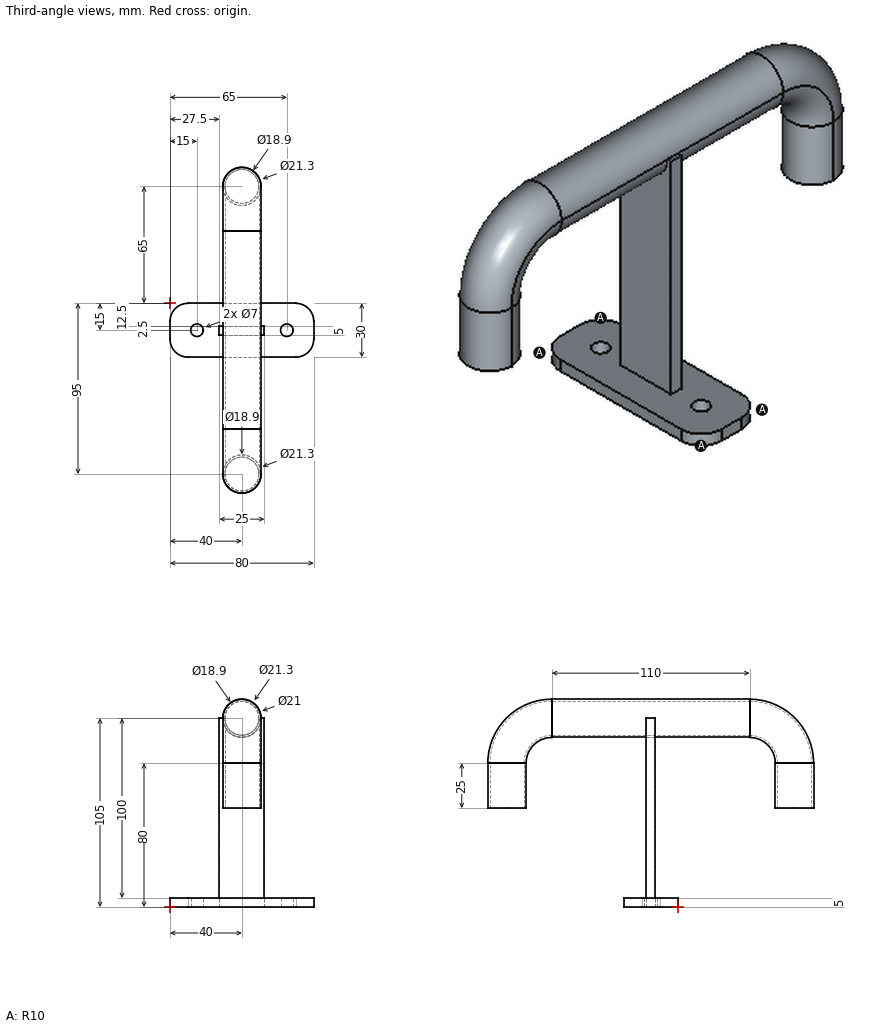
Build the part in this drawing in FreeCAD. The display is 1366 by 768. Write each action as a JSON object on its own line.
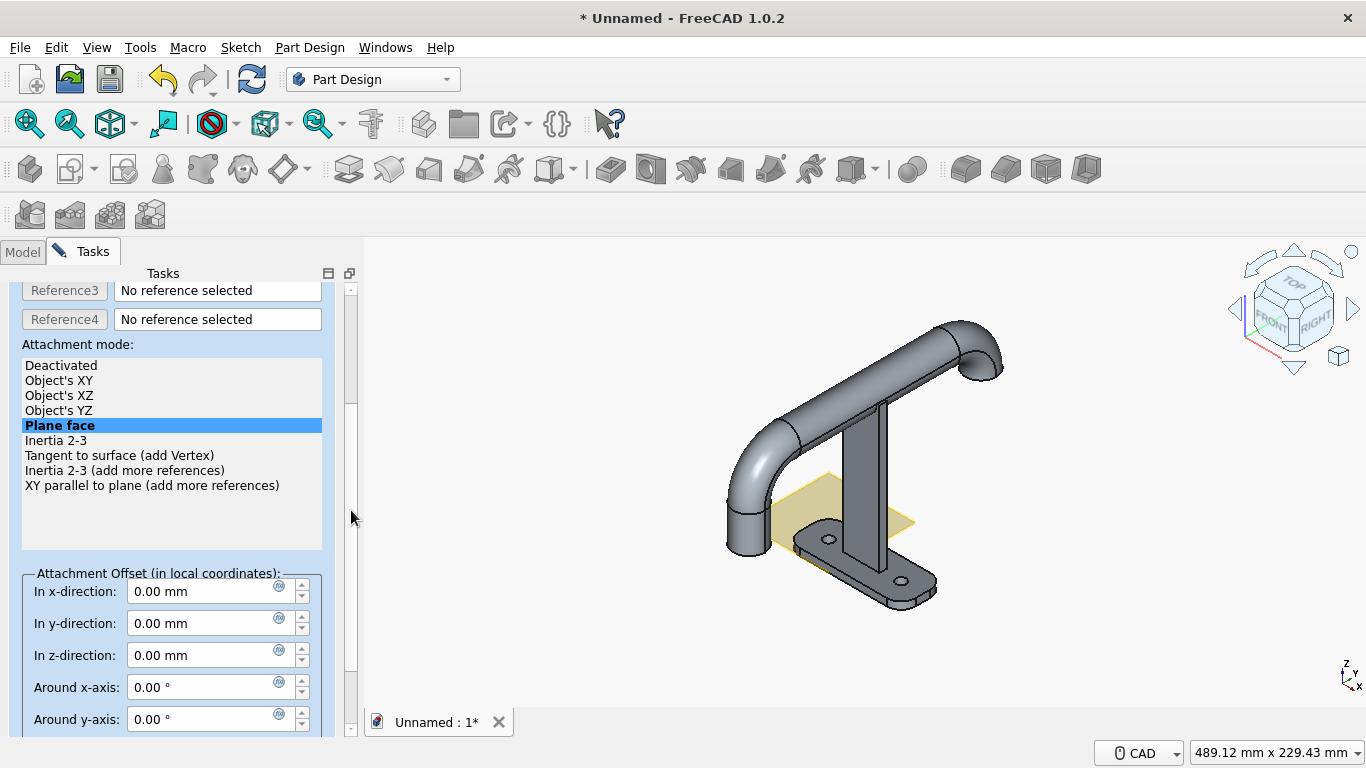
{"action": "triple_click", "coordinate": [210, 655]}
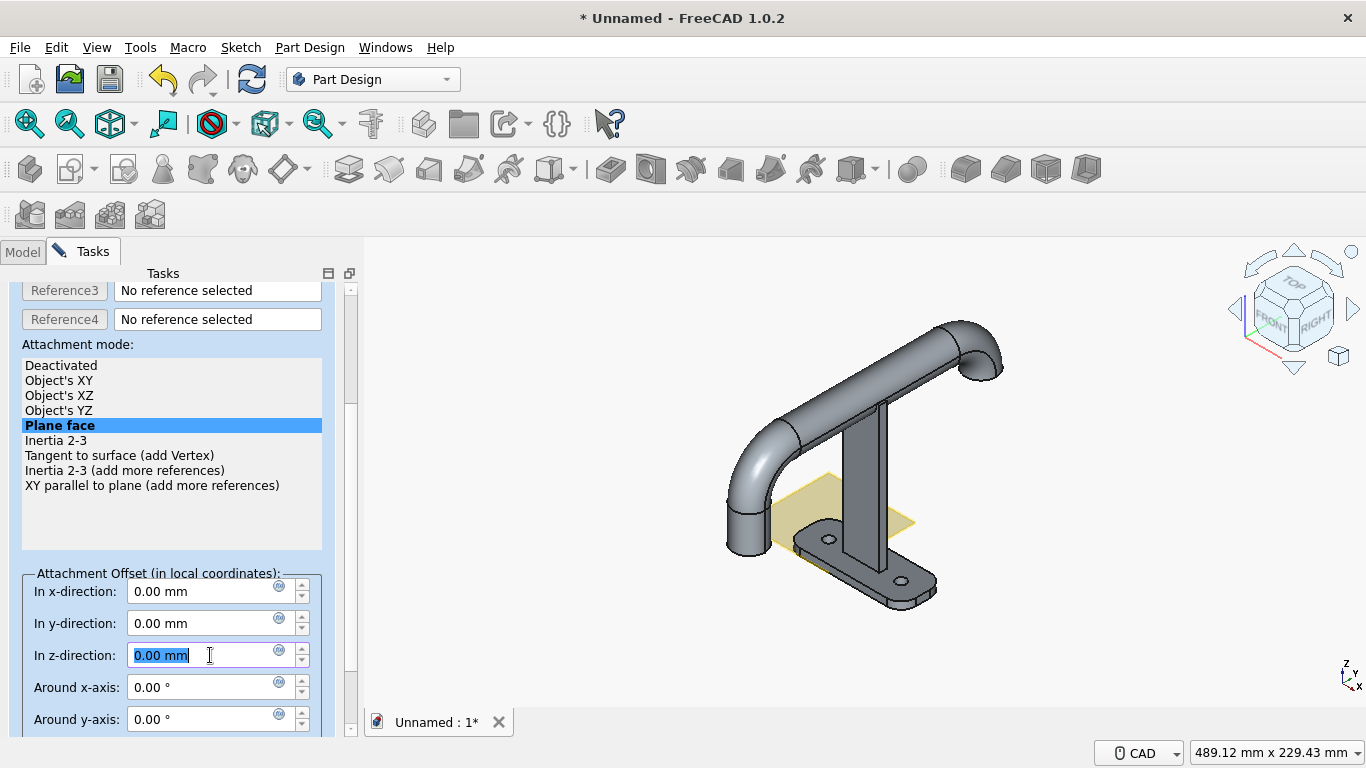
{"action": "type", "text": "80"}
{"action": "key", "text": "Tab"}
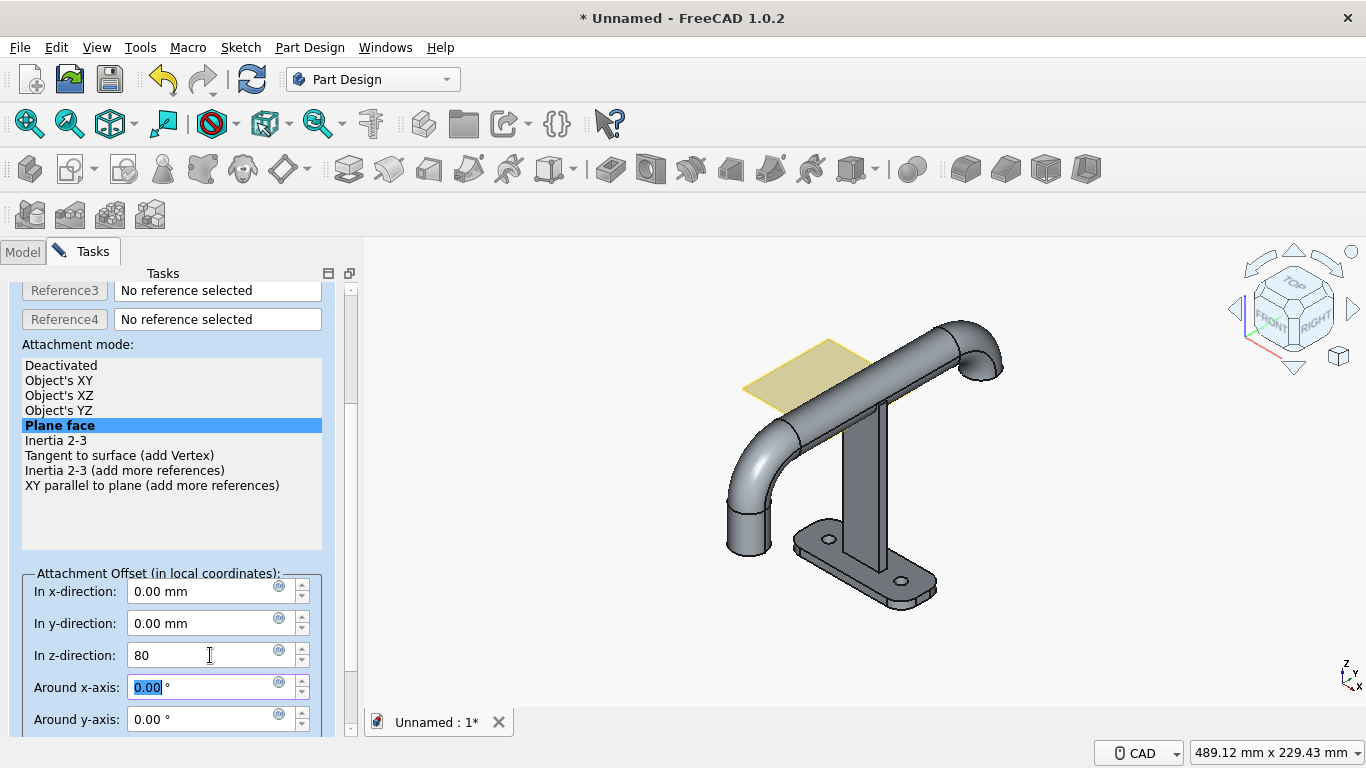
{"action": "scroll", "coordinate": [351, 510], "scroll_direction": "up", "scroll_amount": 4}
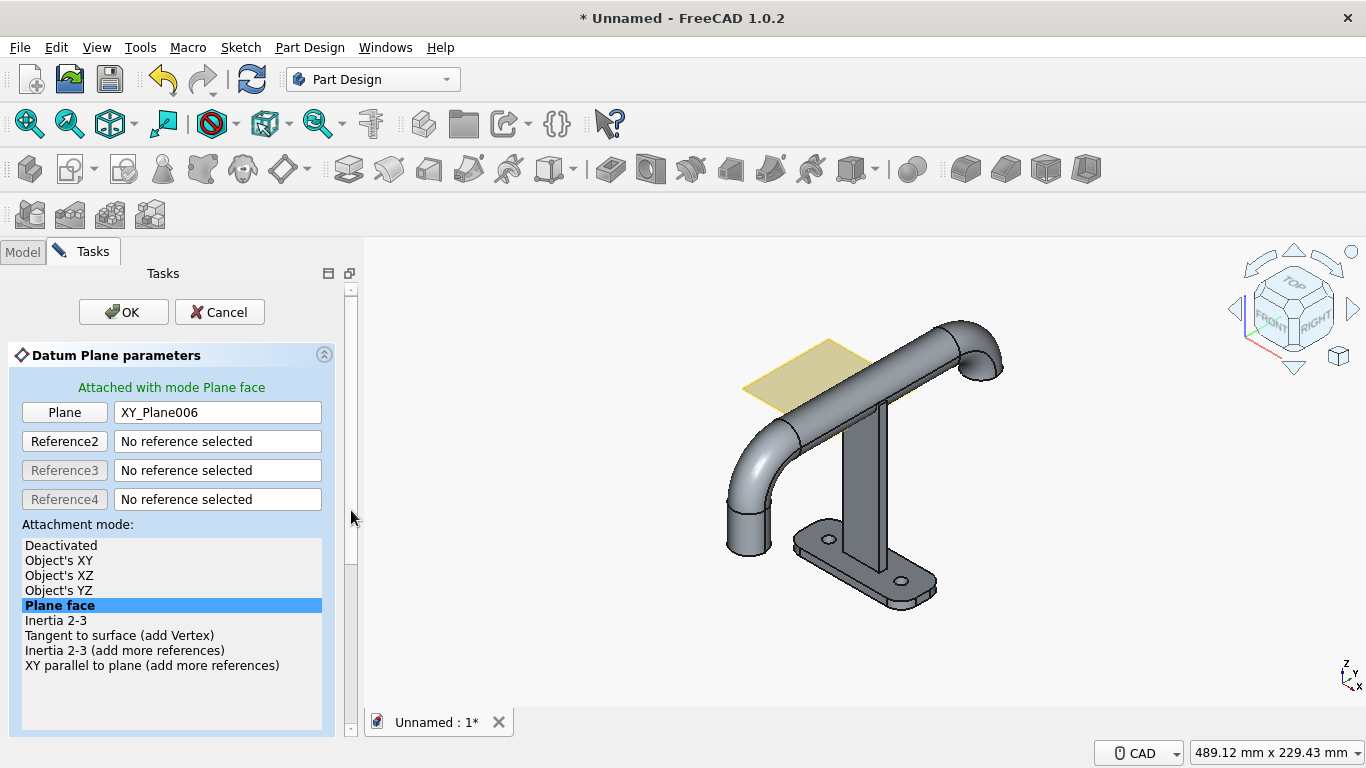
{"action": "left_click", "coordinate": [124, 312]}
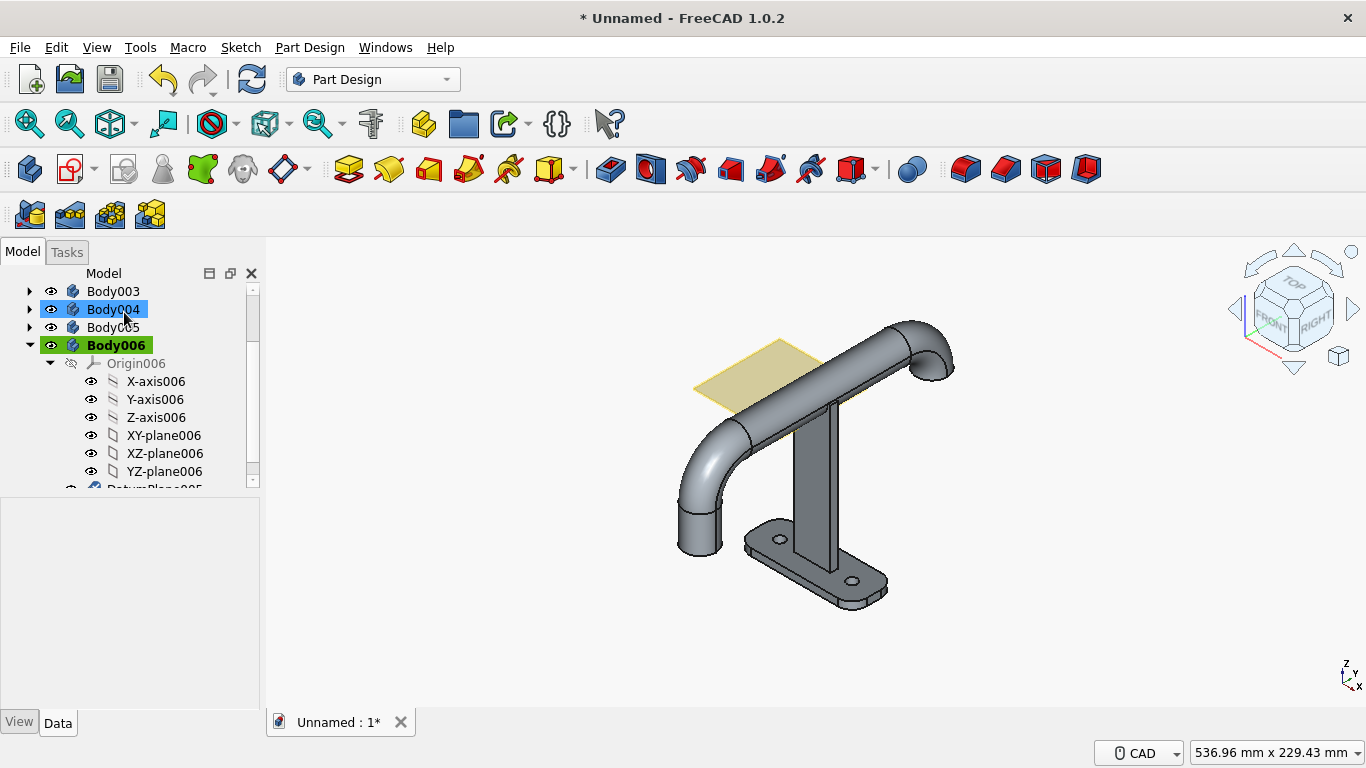
{"action": "scroll", "coordinate": [120, 377], "scroll_direction": "down", "scroll_amount": 3}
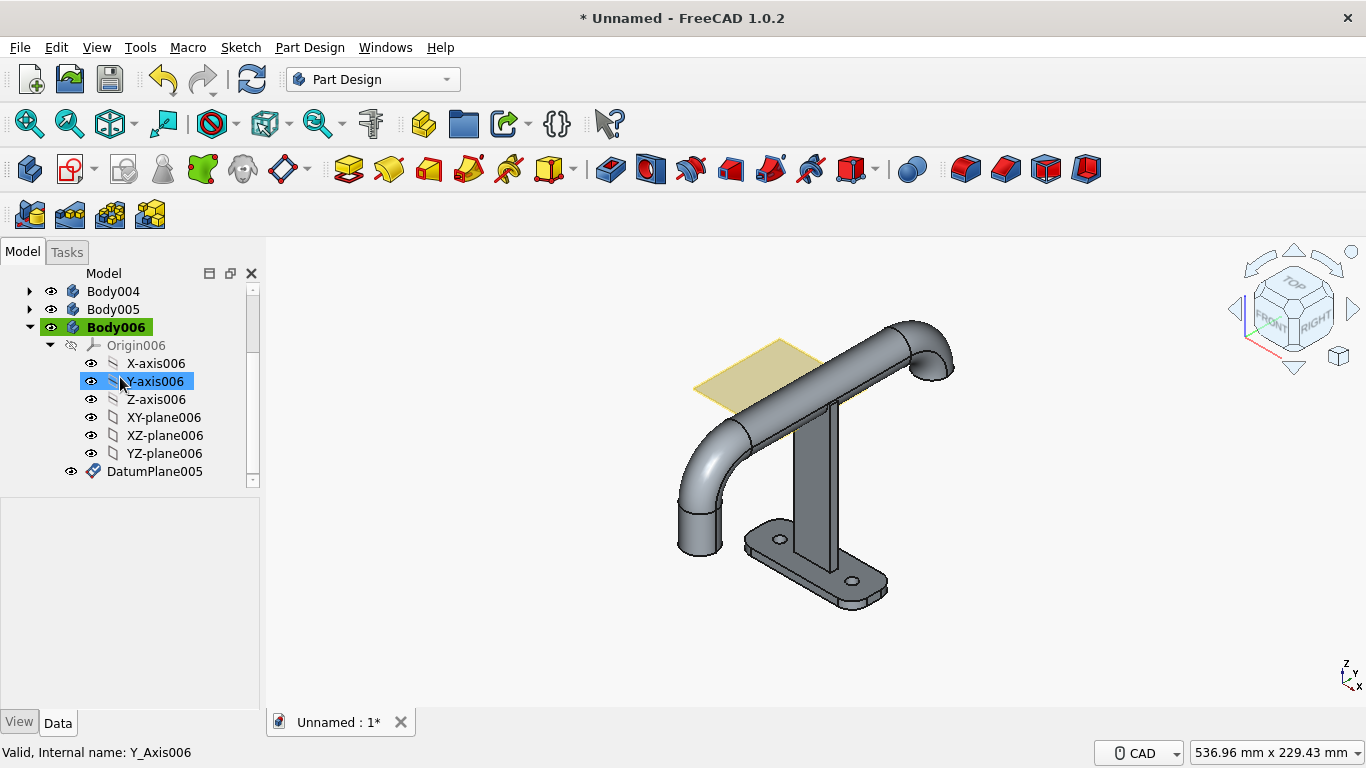
{"action": "left_click", "coordinate": [116, 471]}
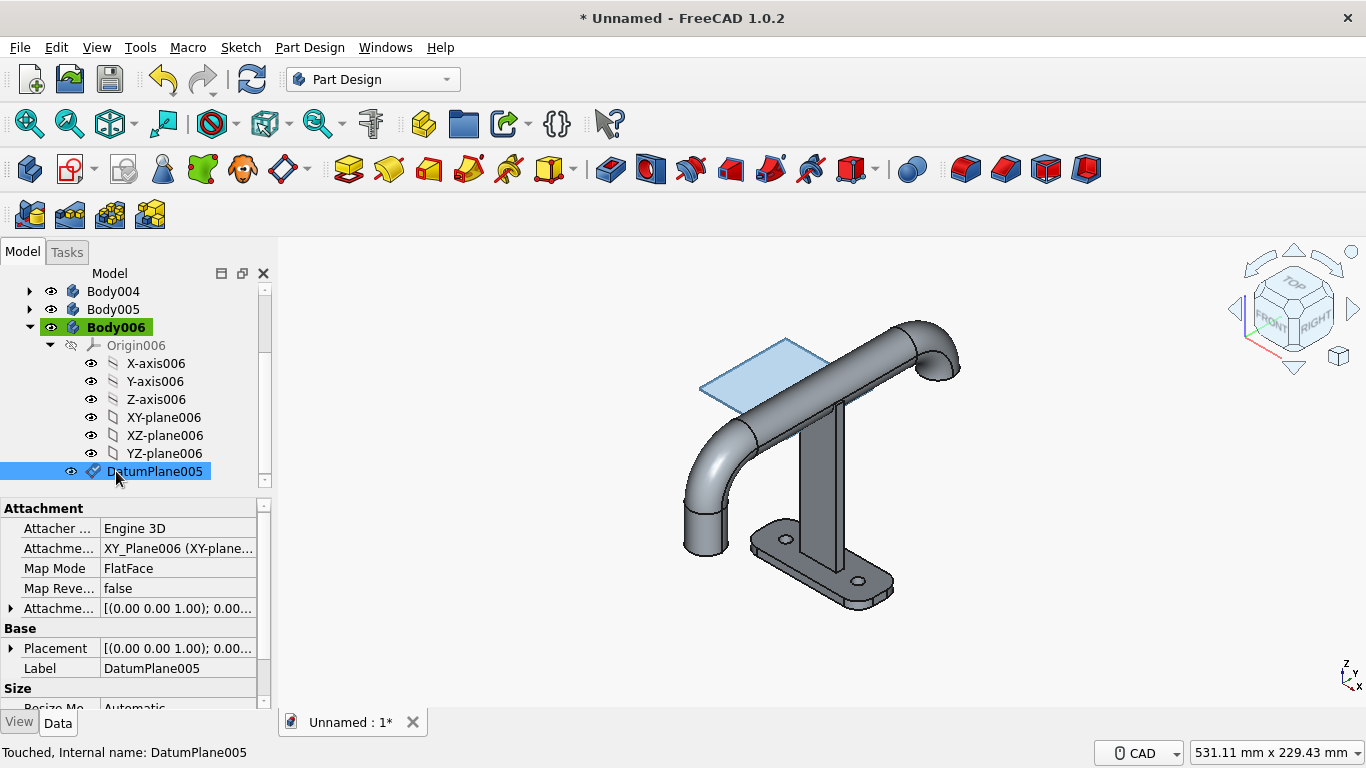
{"action": "left_click", "coordinate": [70, 170]}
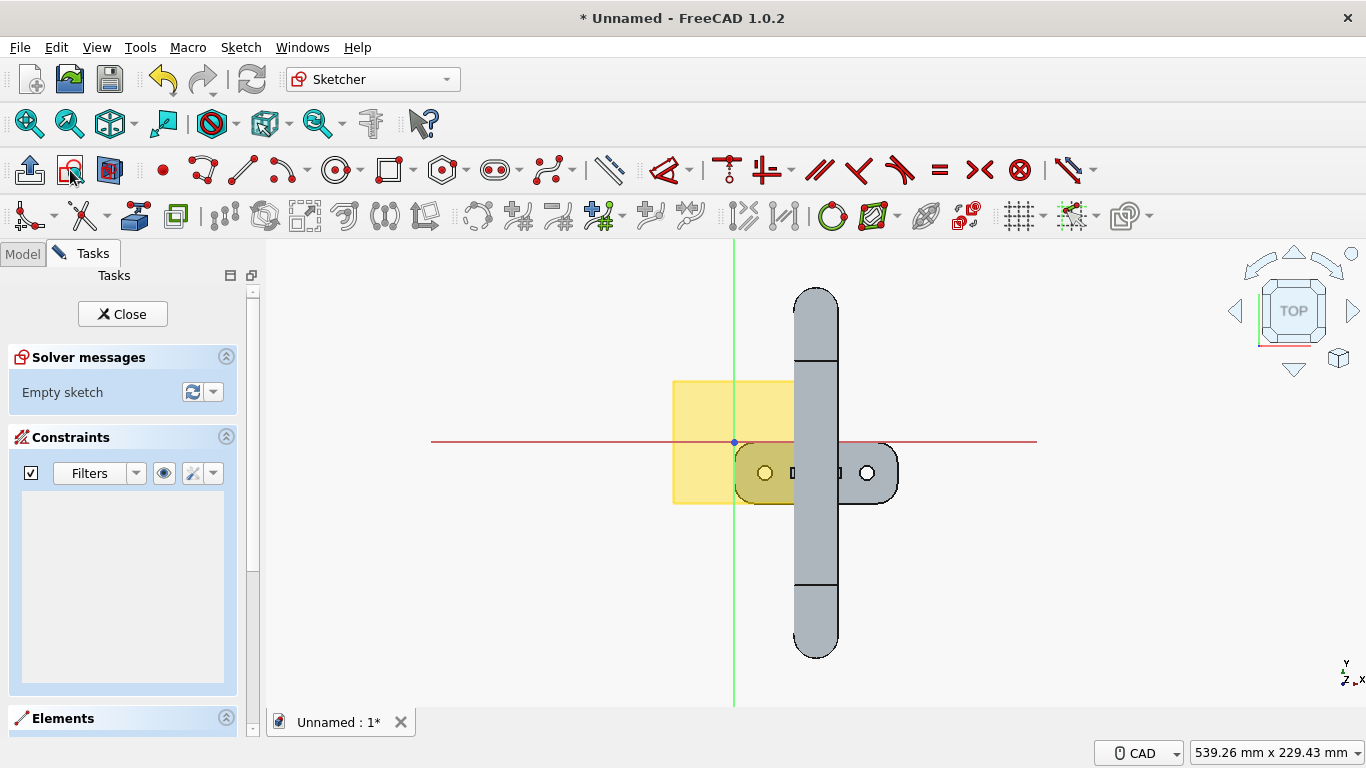
{"action": "scroll", "coordinate": [827, 284], "scroll_direction": "up", "scroll_amount": 10}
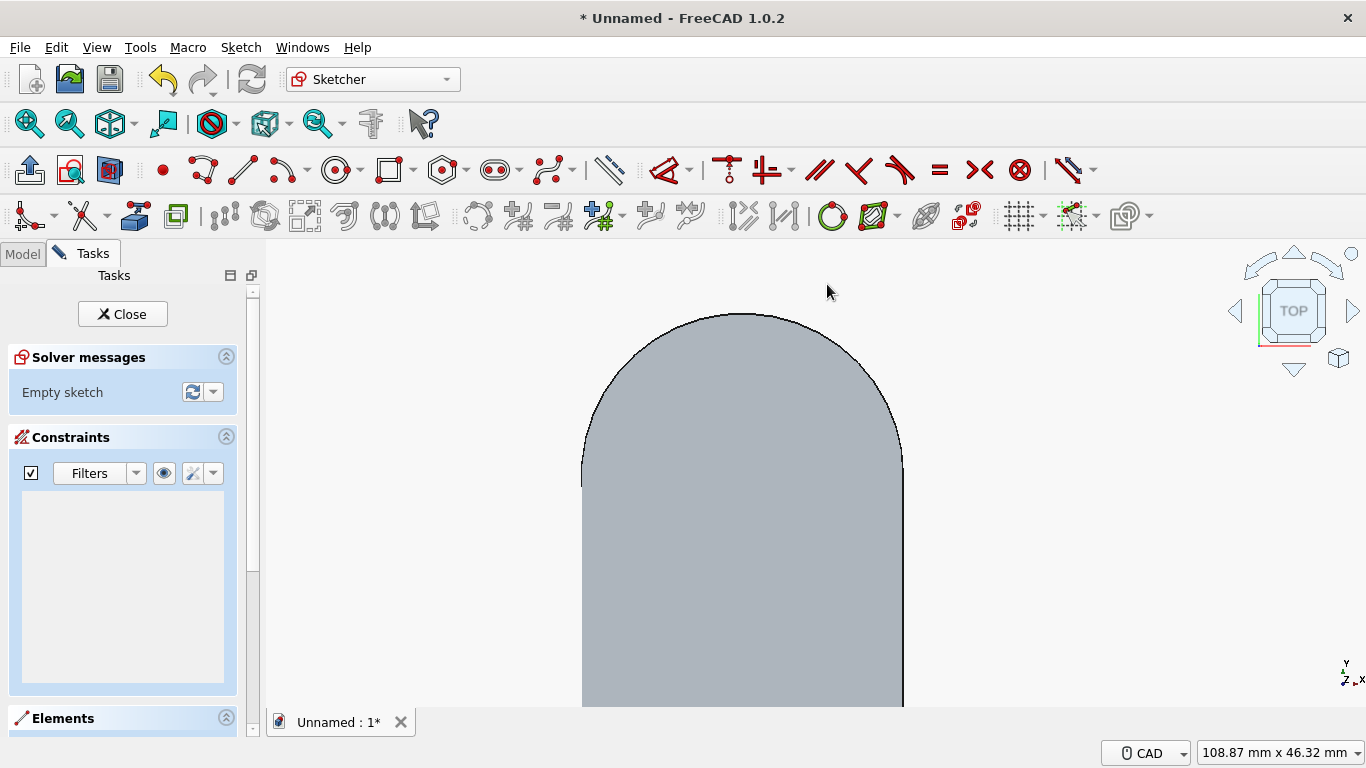
{"action": "left_click", "coordinate": [336, 170]}